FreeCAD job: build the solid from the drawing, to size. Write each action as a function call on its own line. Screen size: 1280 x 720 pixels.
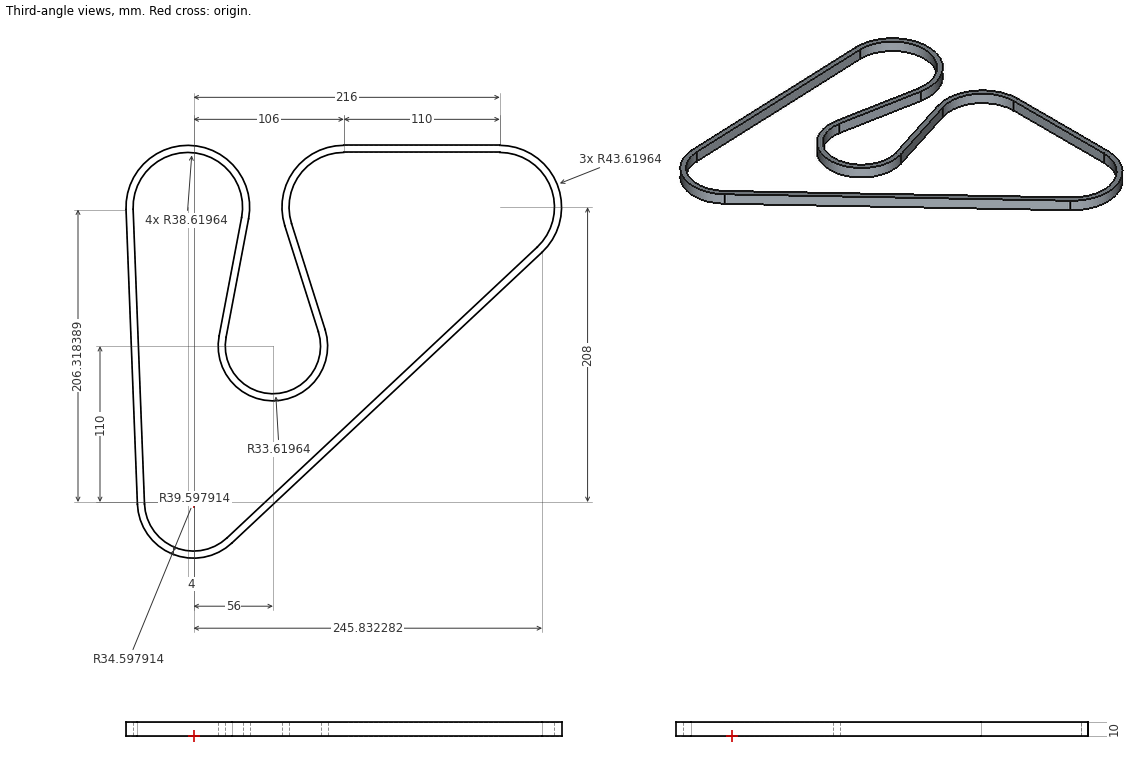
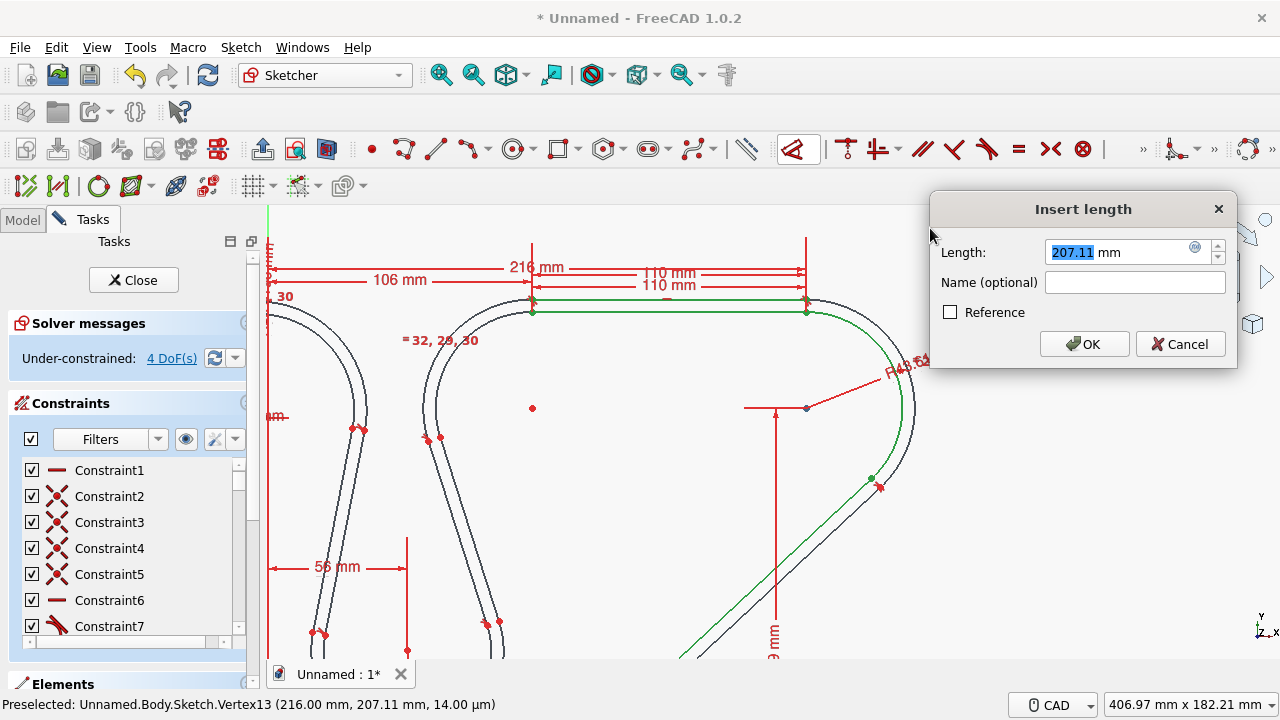
text(208)
key(Return)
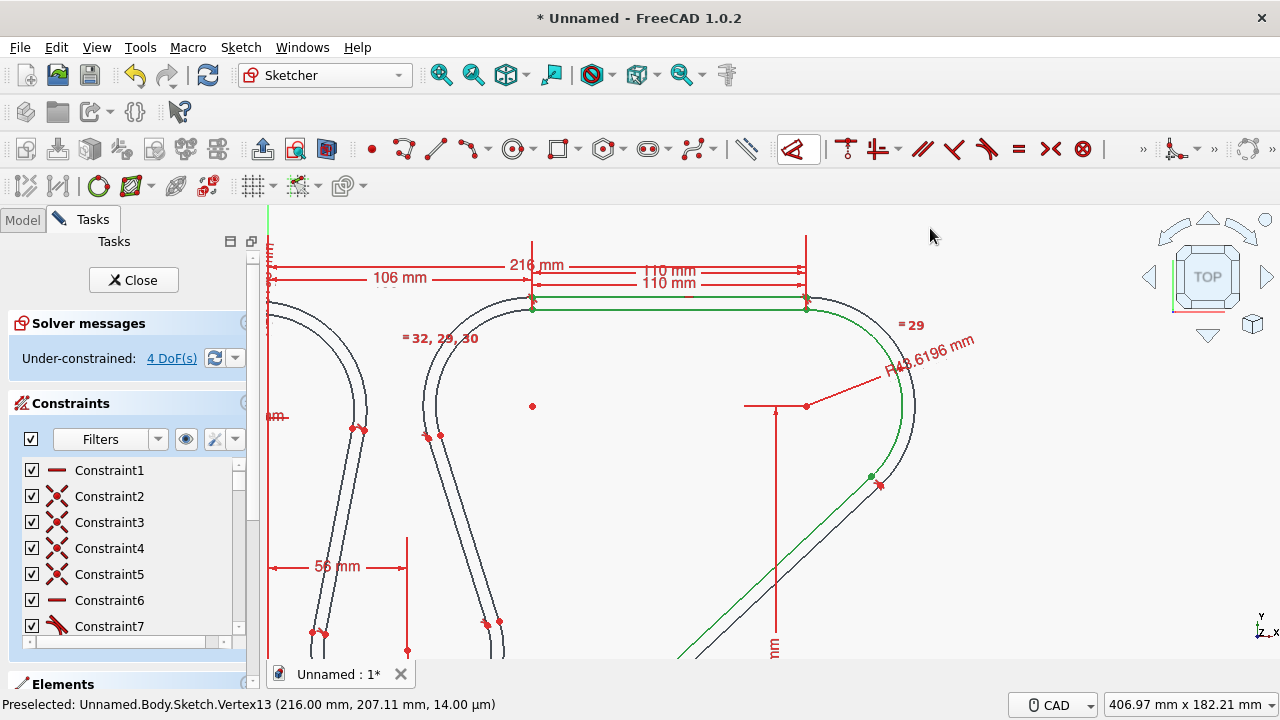
scroll(807, 301, down, 5)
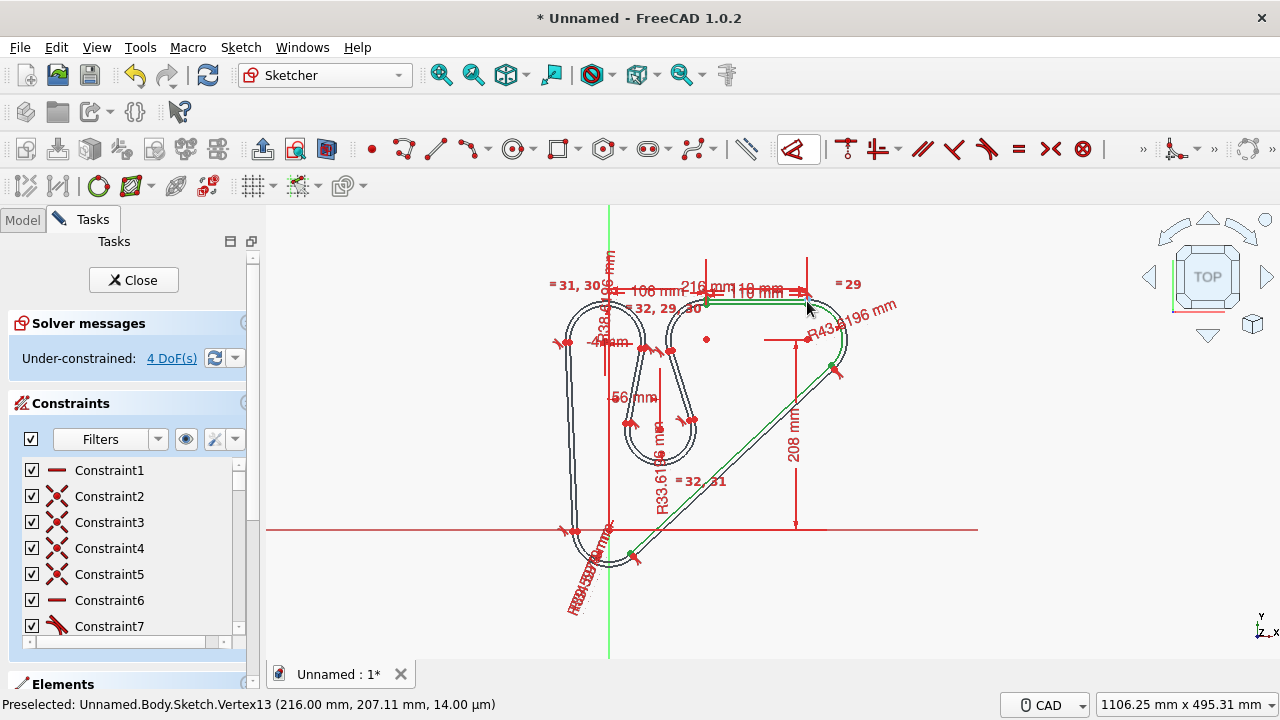
click(660, 430)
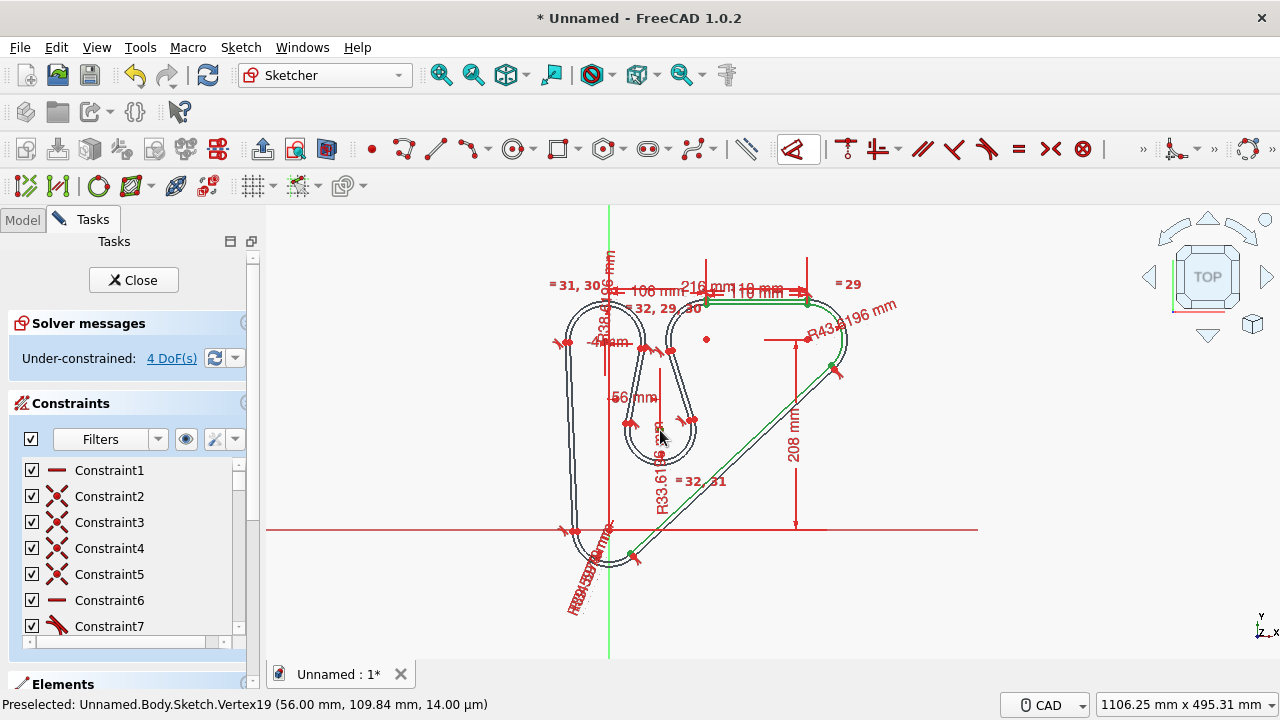
click(814, 150)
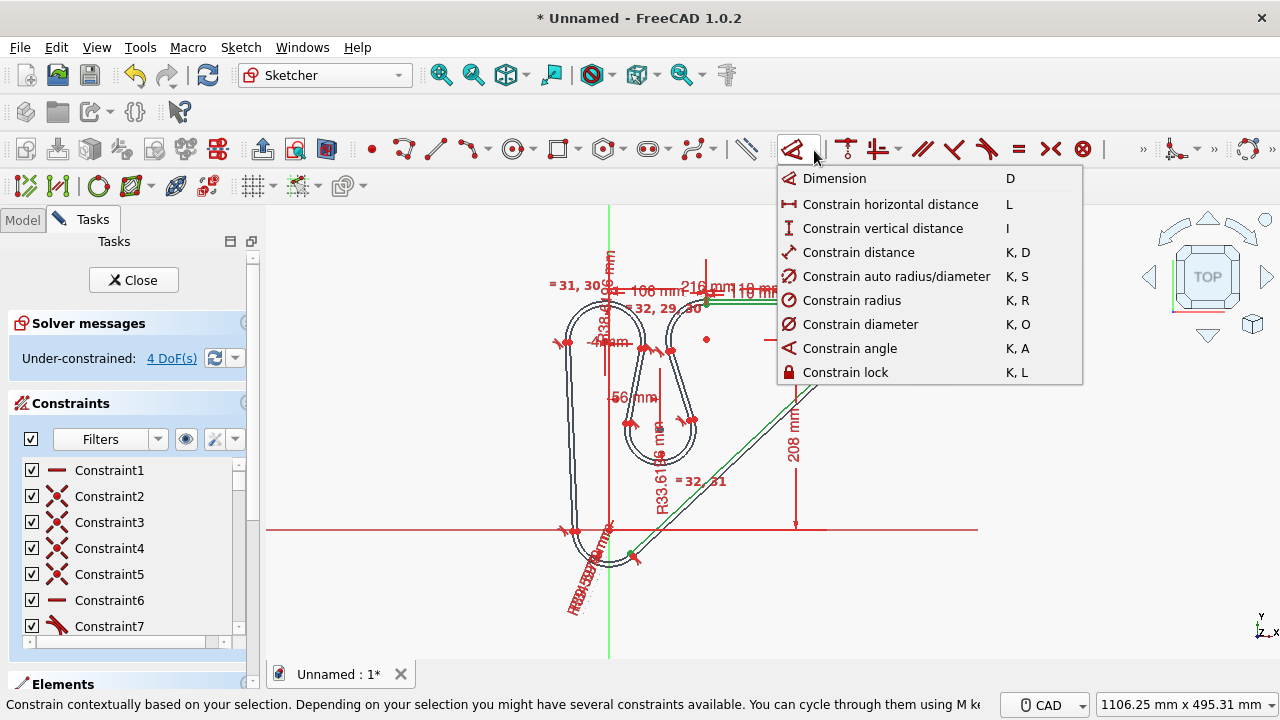
click(930, 228)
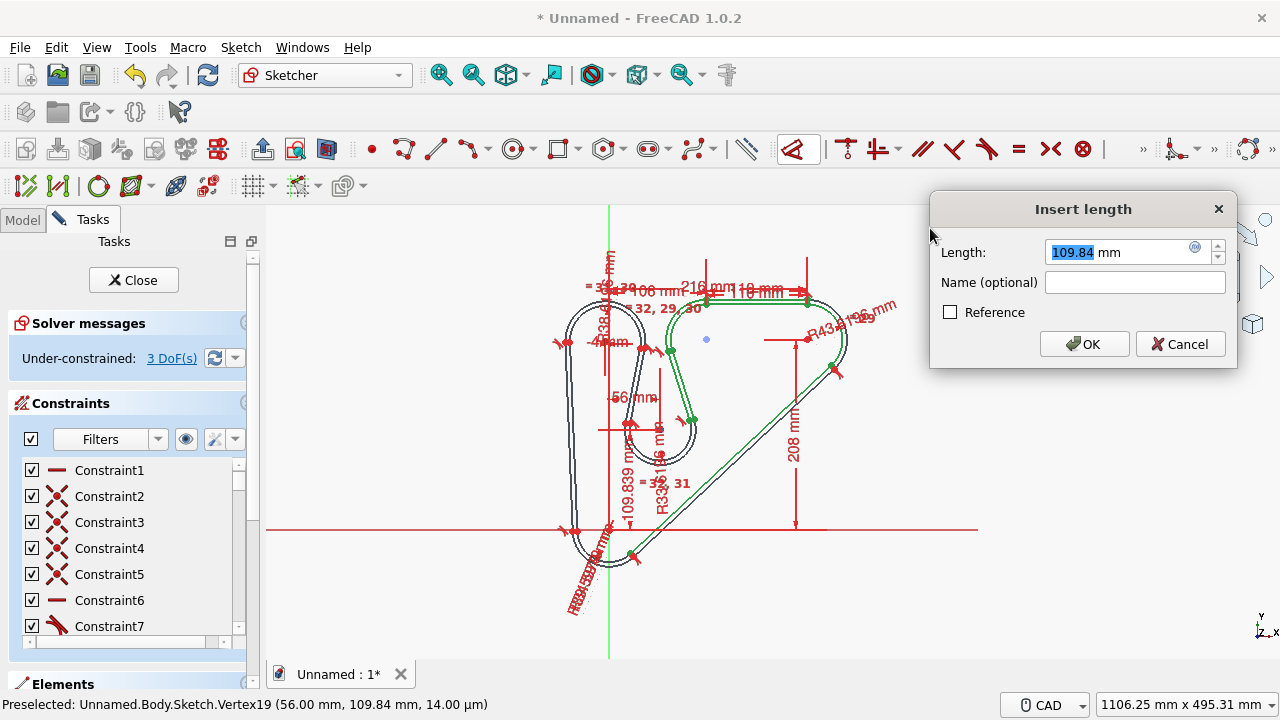
text(110)
key(Return)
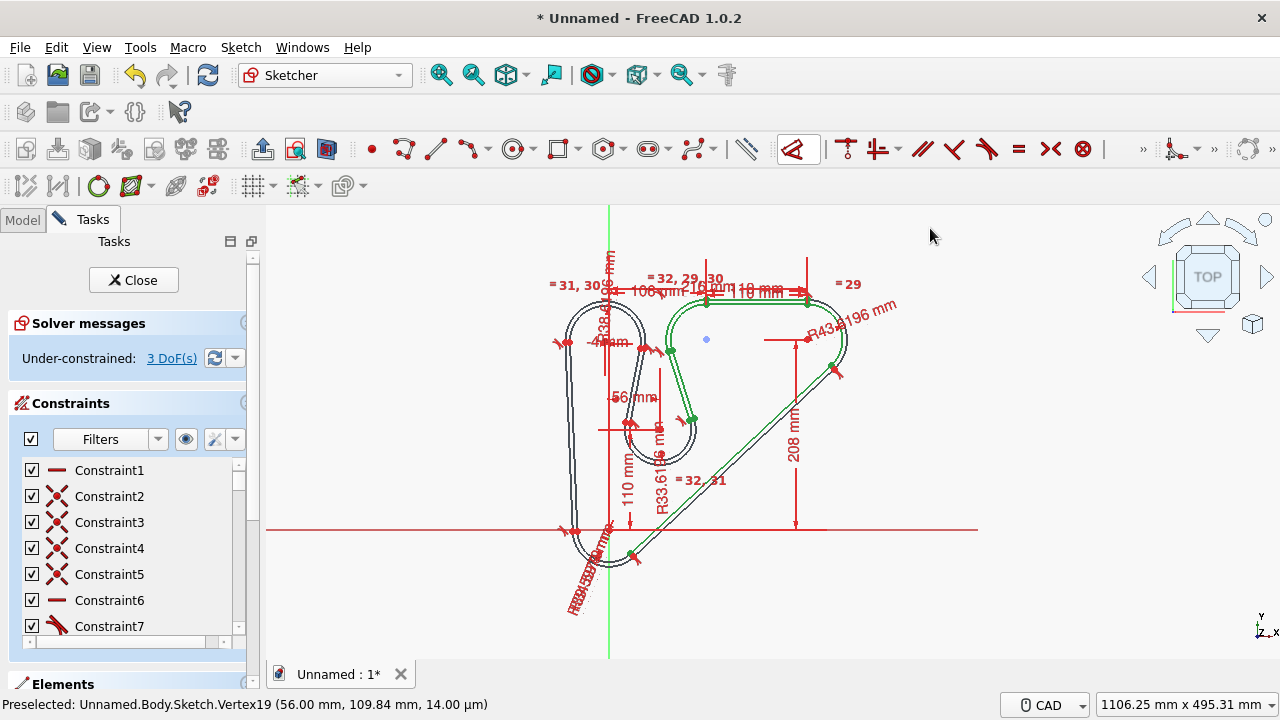
click(605, 341)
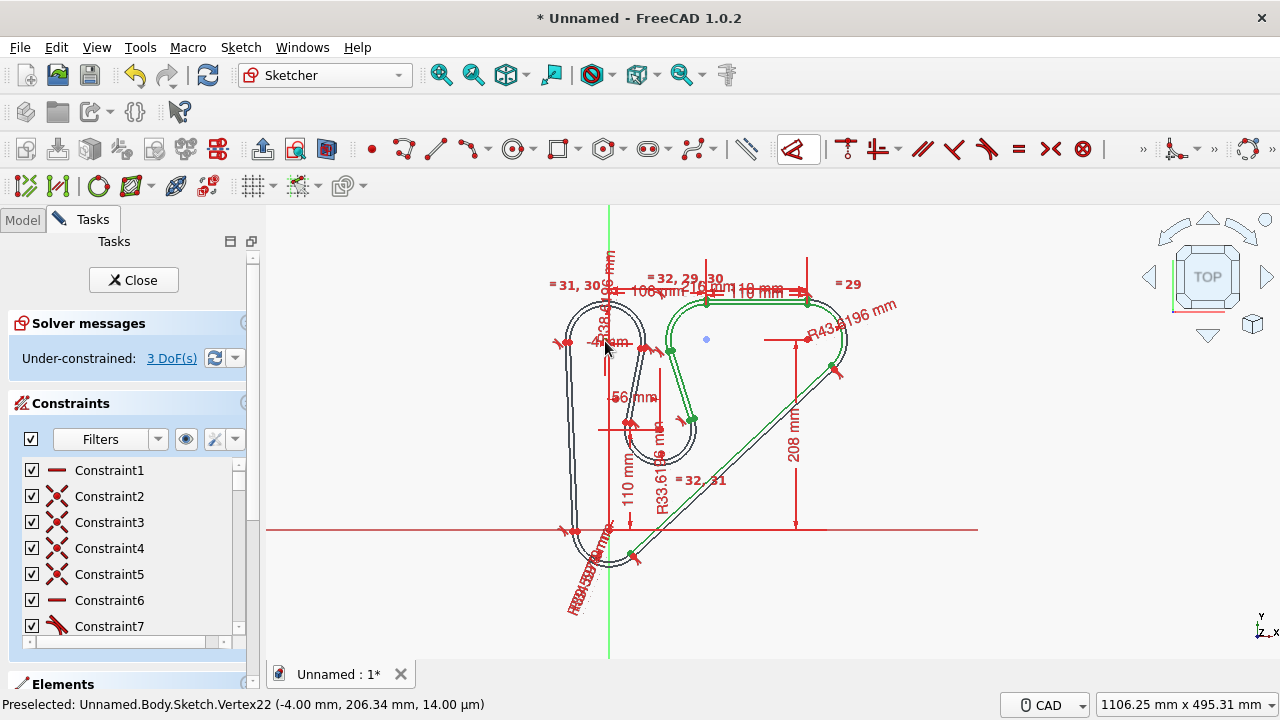
key(i)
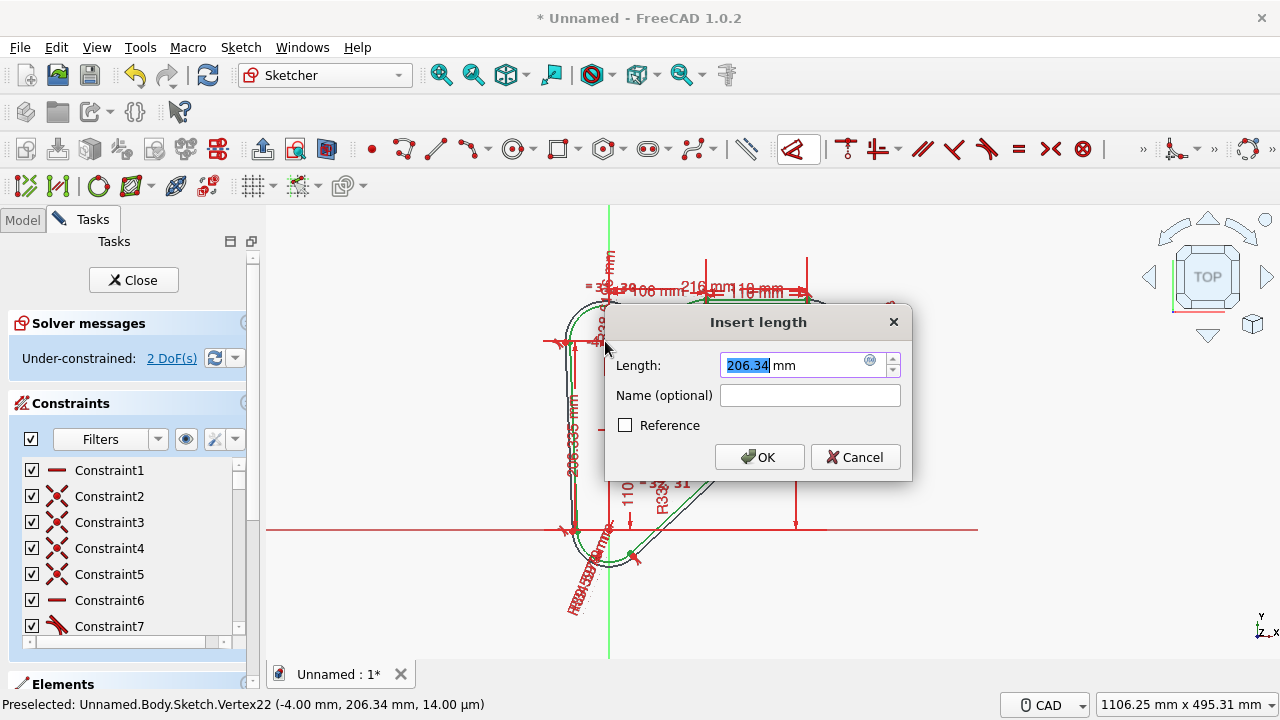
text(208)
key(Return)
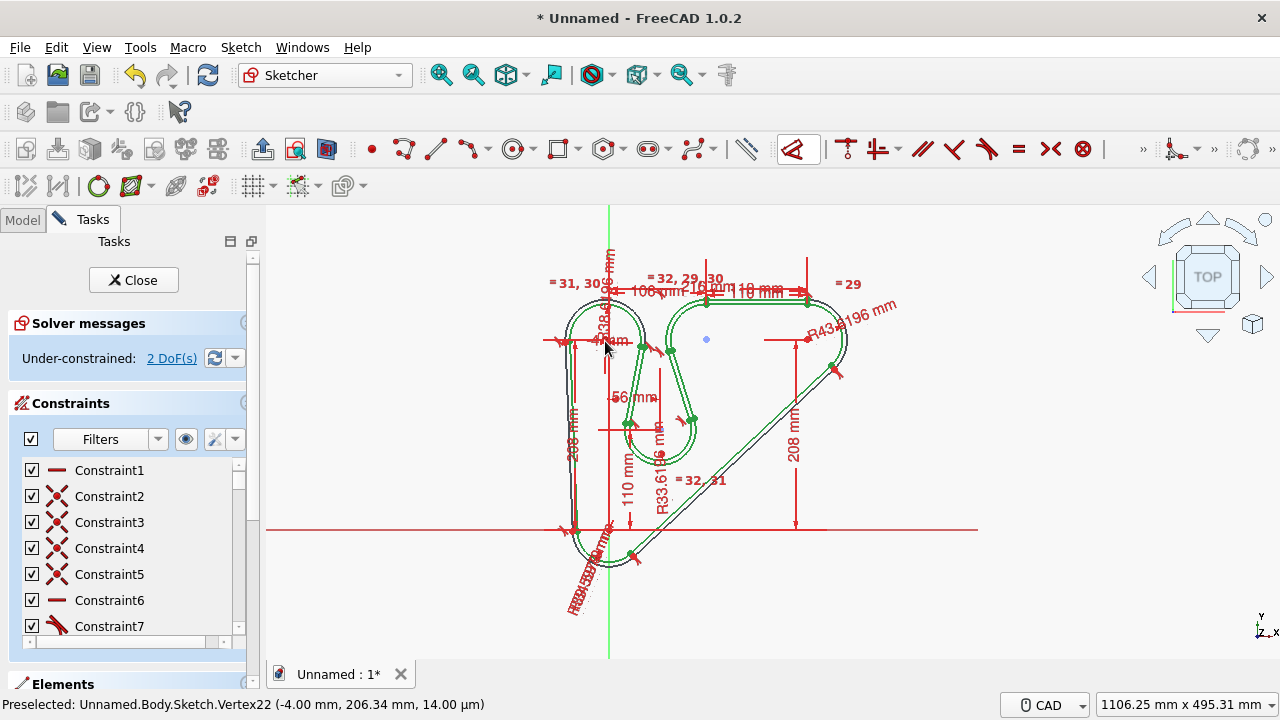
scroll(834, 369, up, 5)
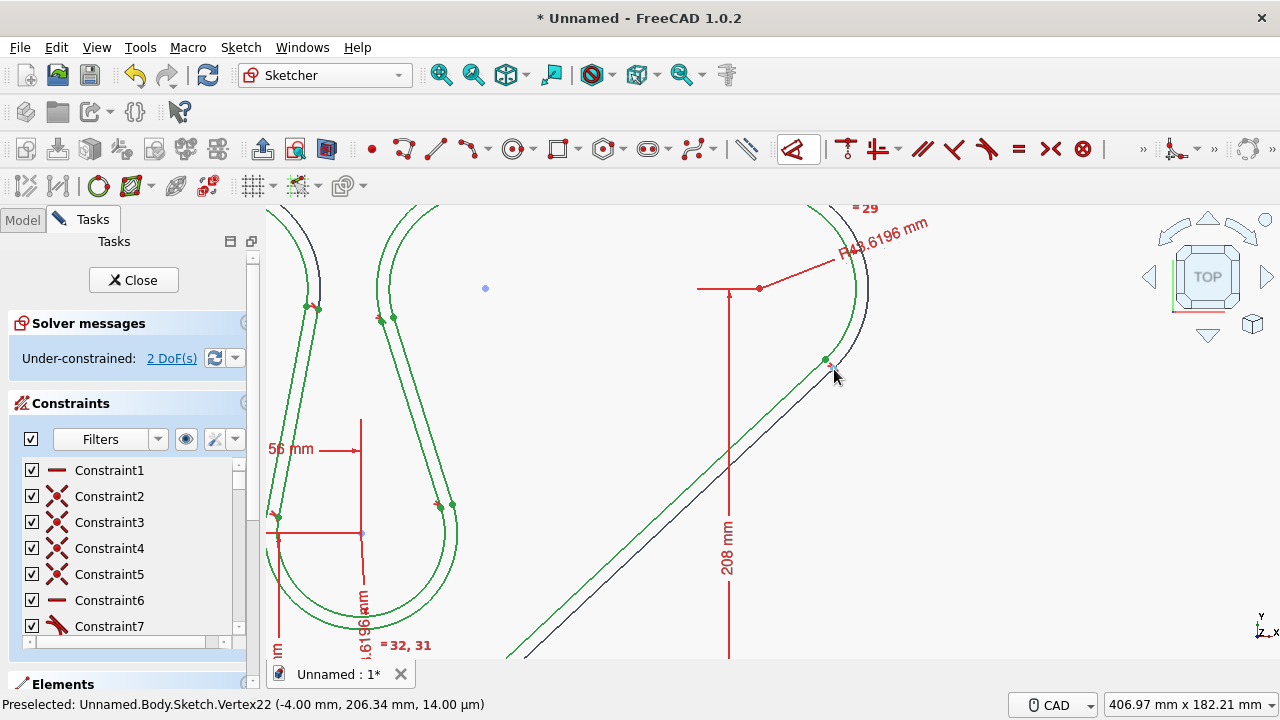
click(834, 369)